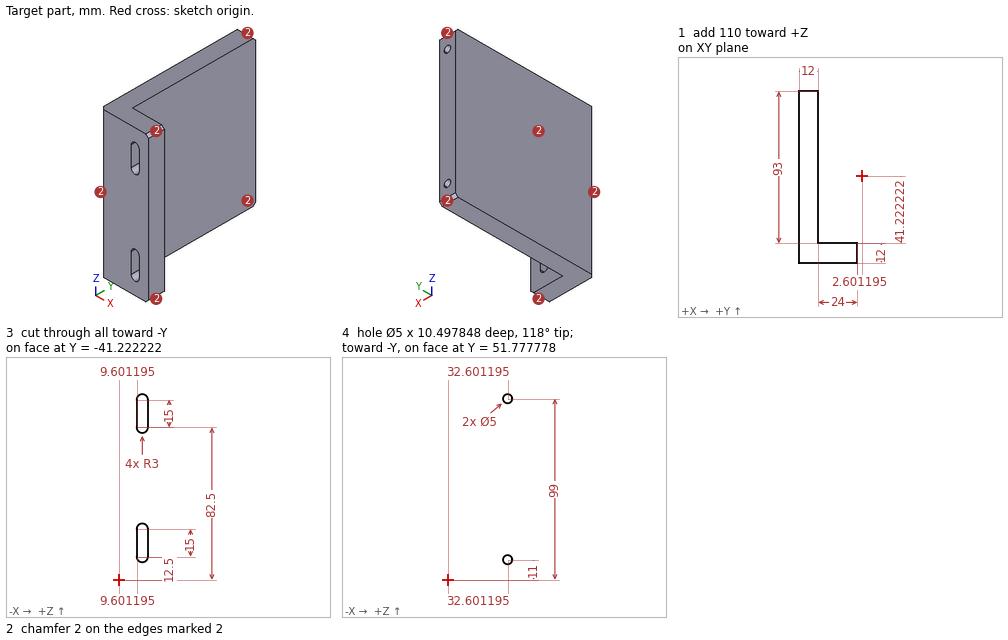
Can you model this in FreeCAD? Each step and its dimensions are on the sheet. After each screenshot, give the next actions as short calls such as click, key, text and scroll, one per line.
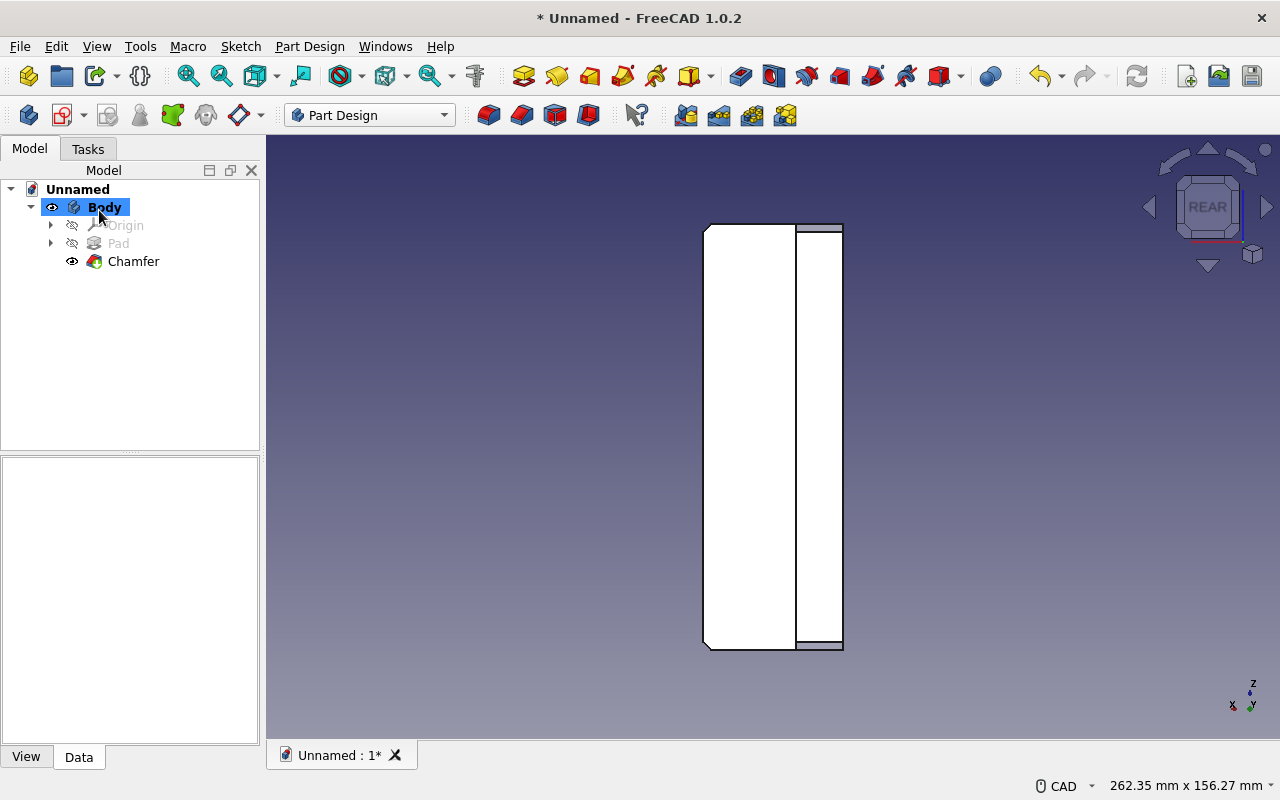
click(750, 315)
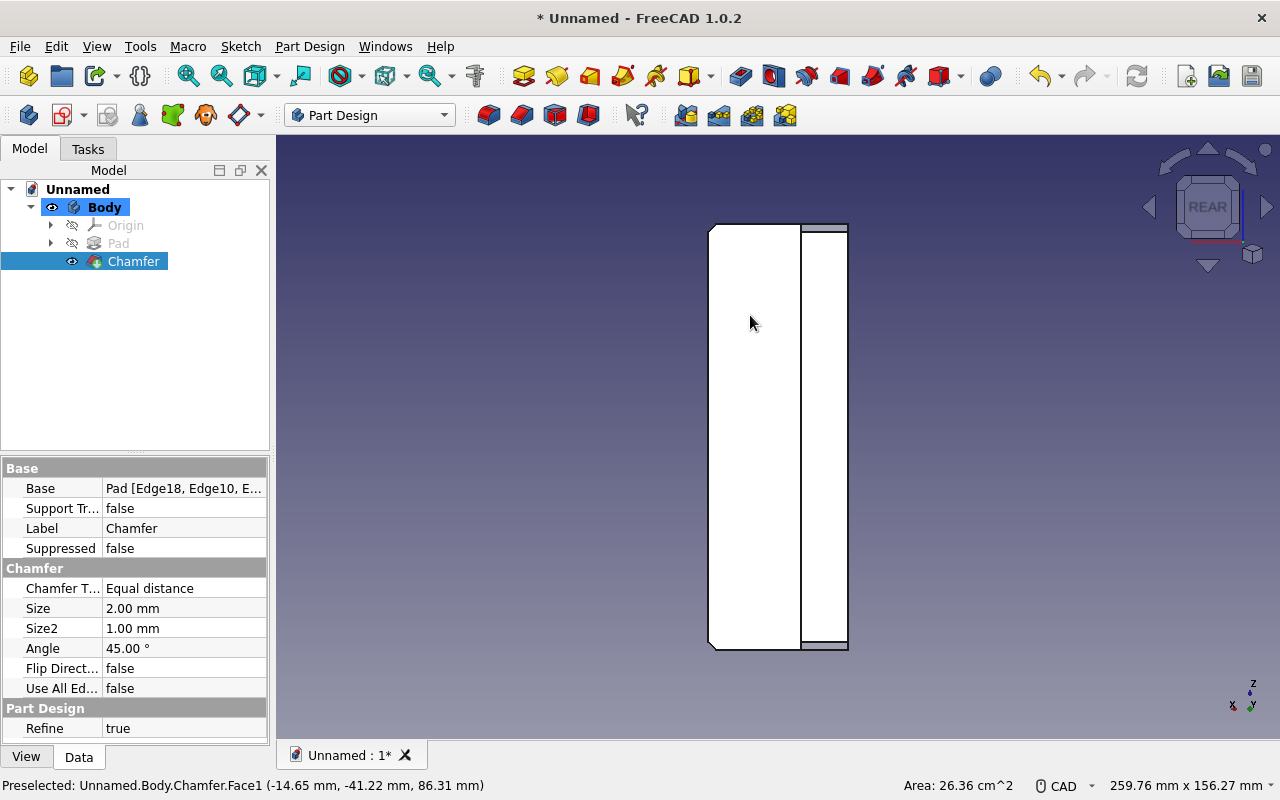
click(62, 116)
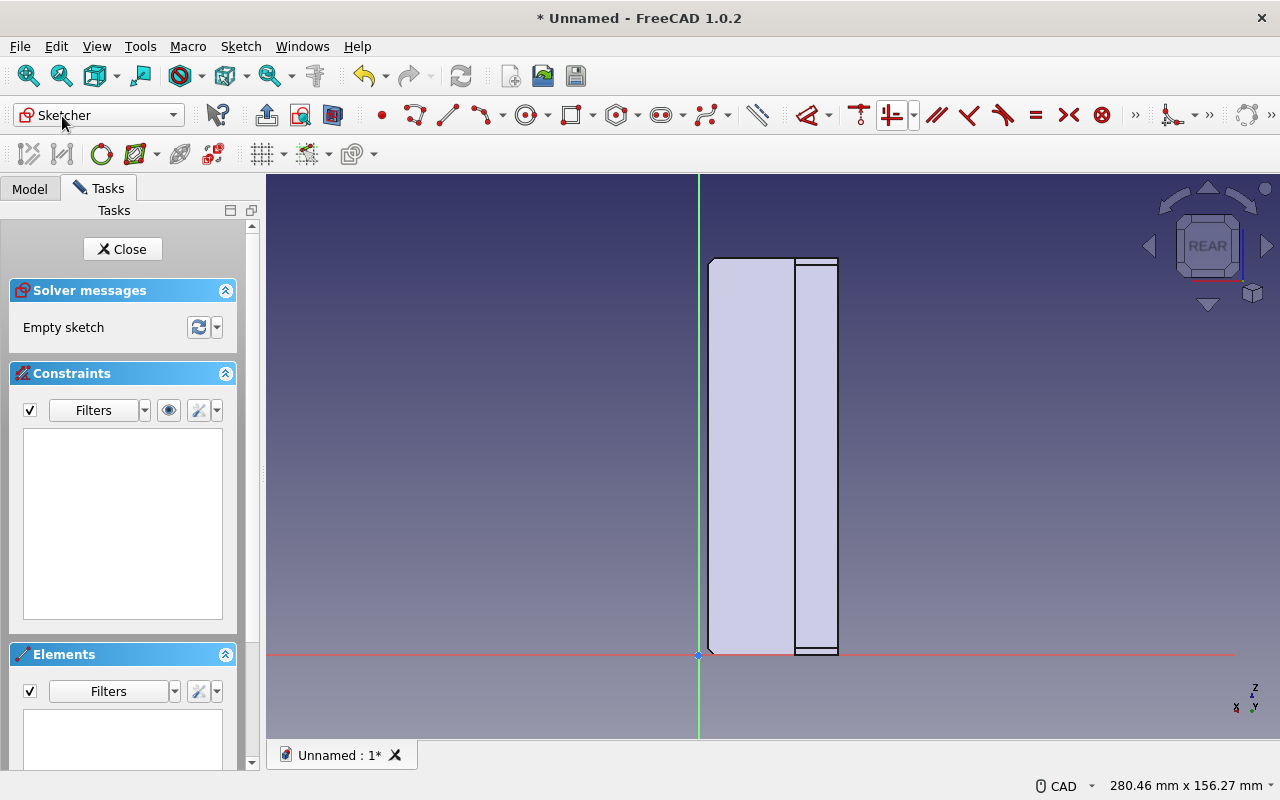
click(333, 116)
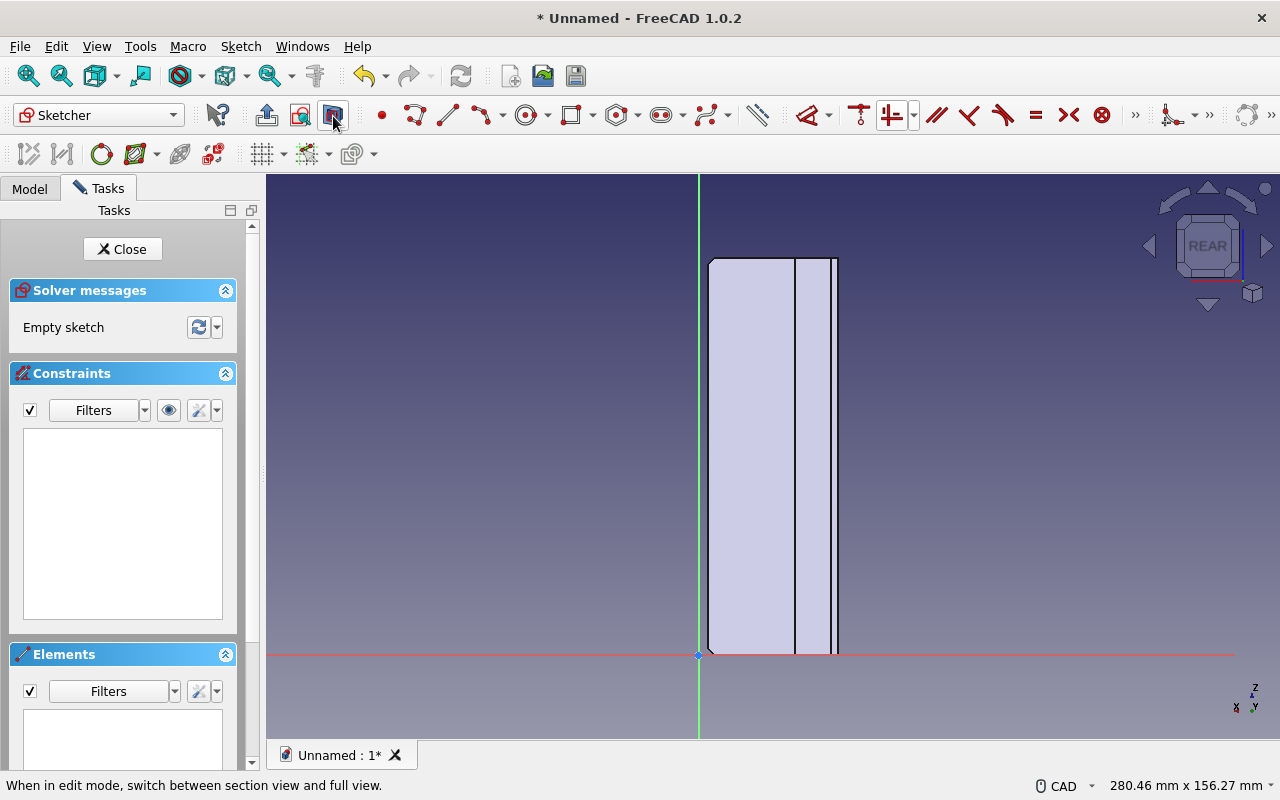
click(660, 116)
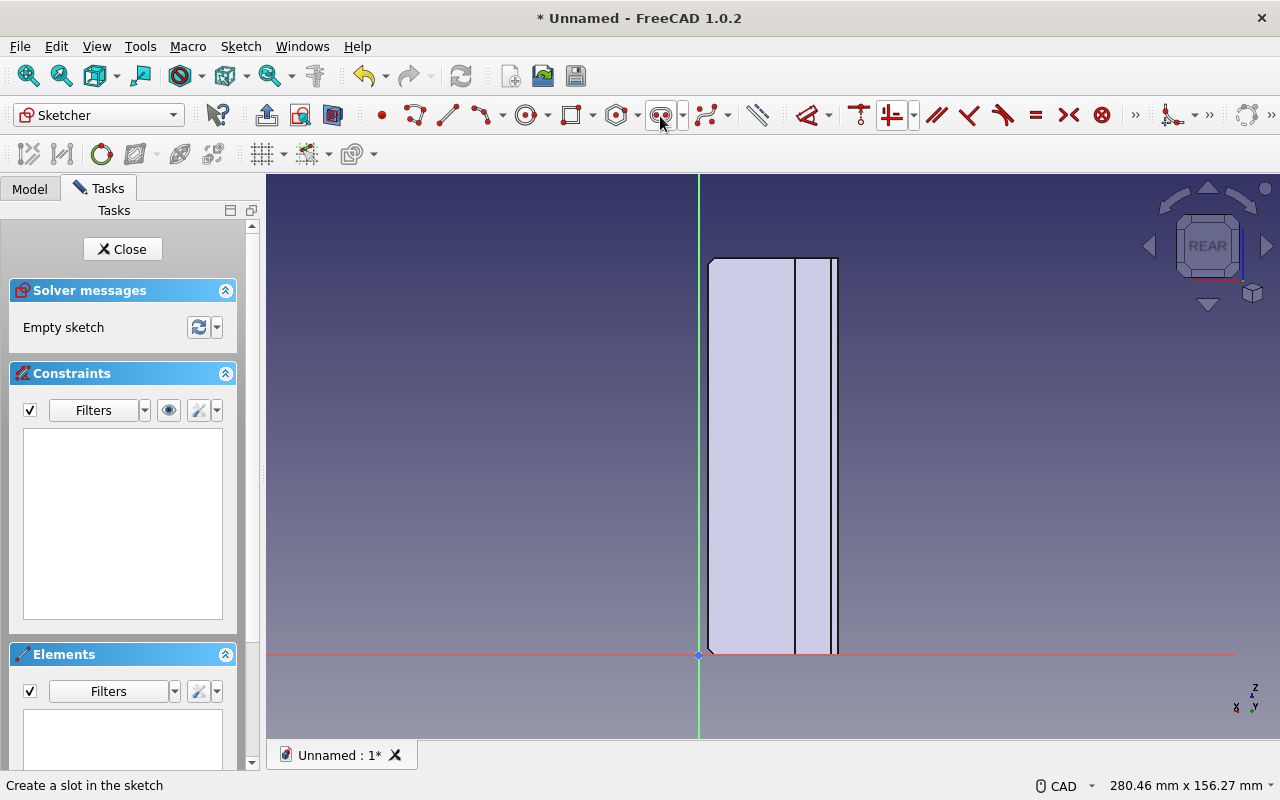
scroll(744, 357, up, 4)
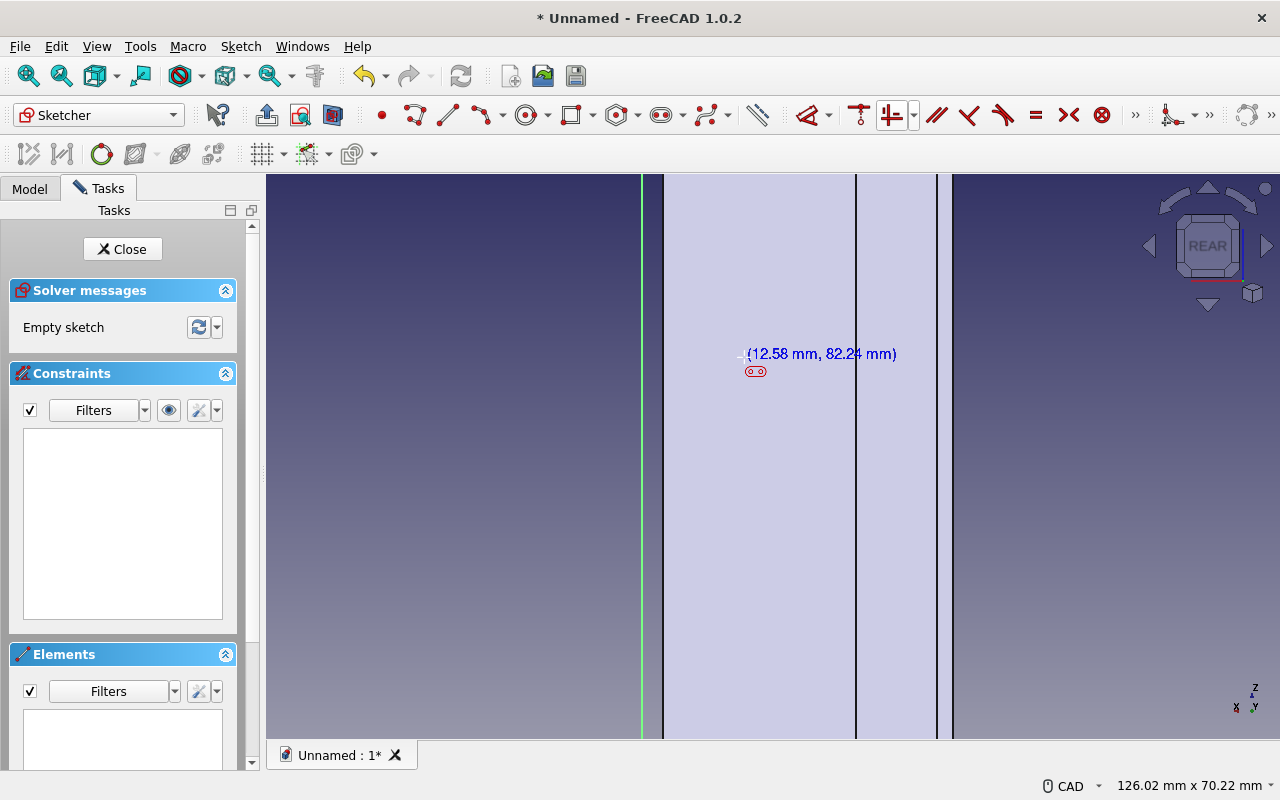
click(744, 357)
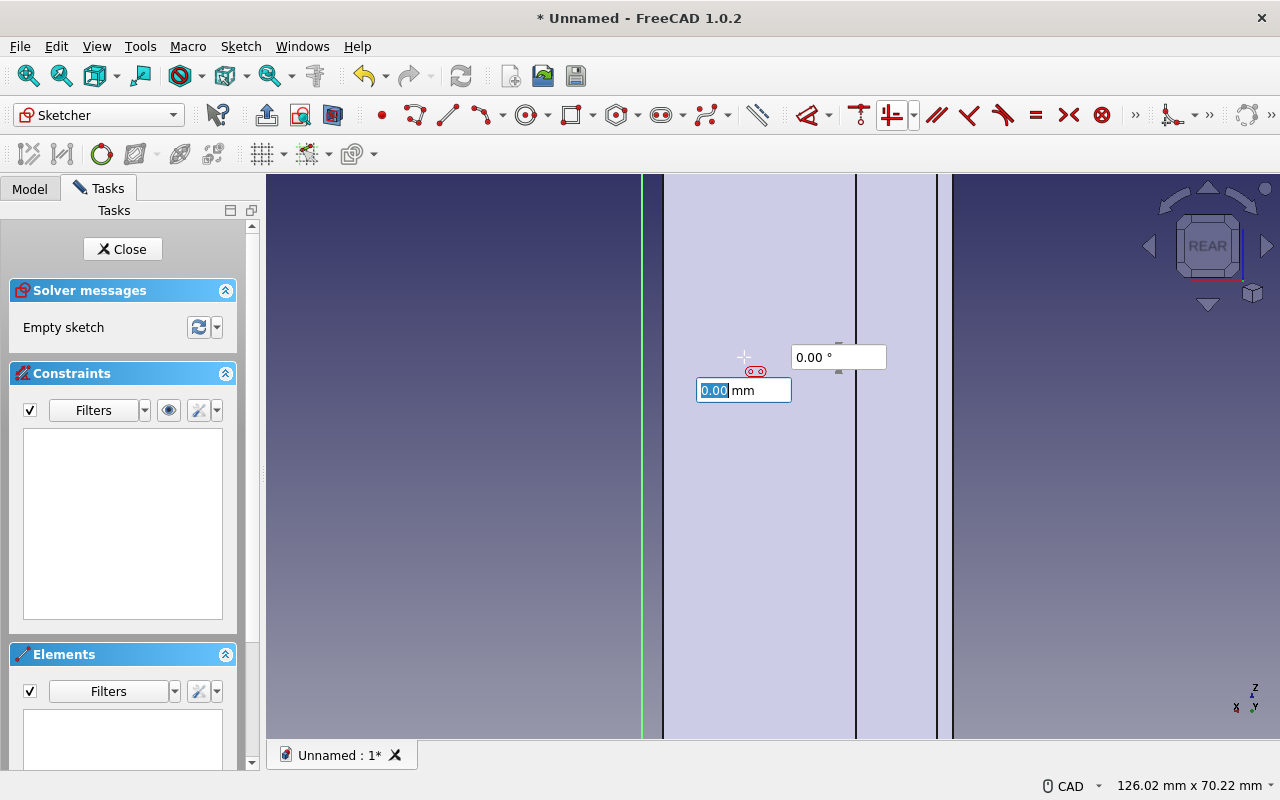
click(744, 236)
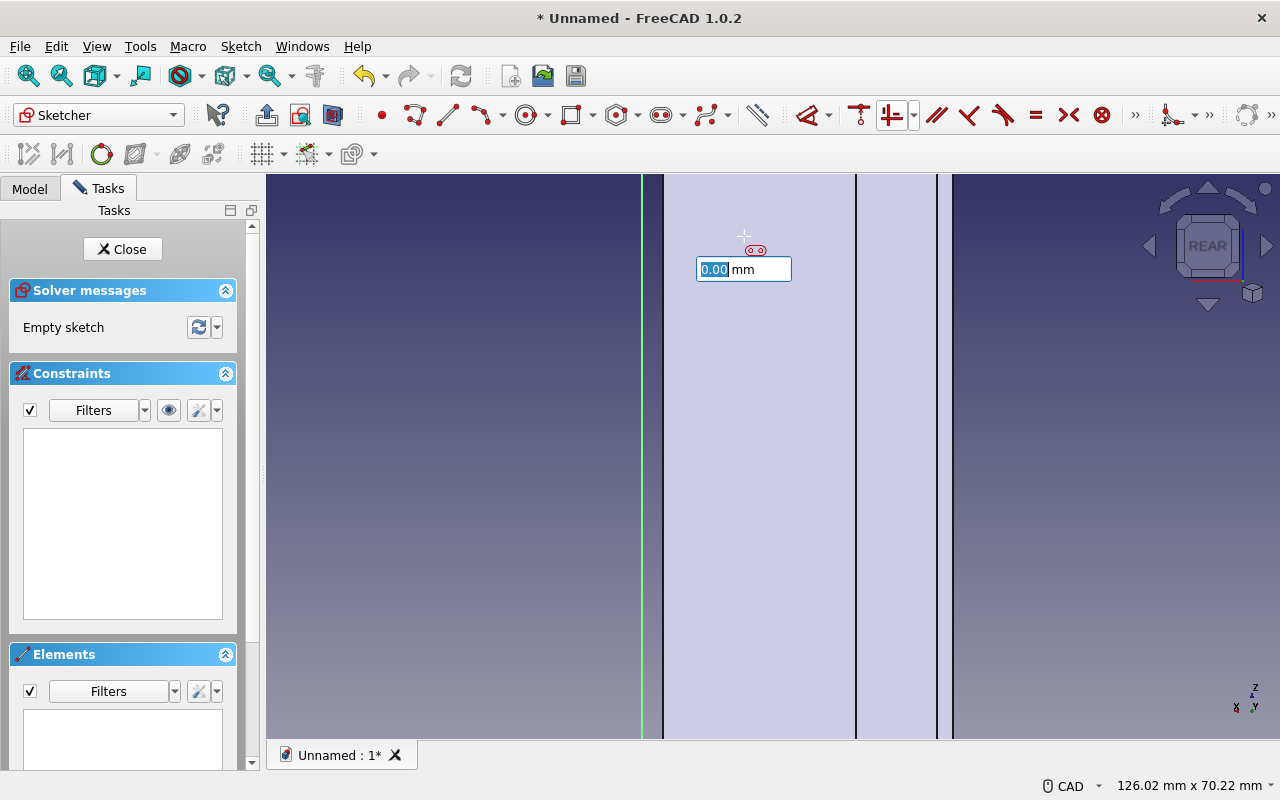
click(768, 296)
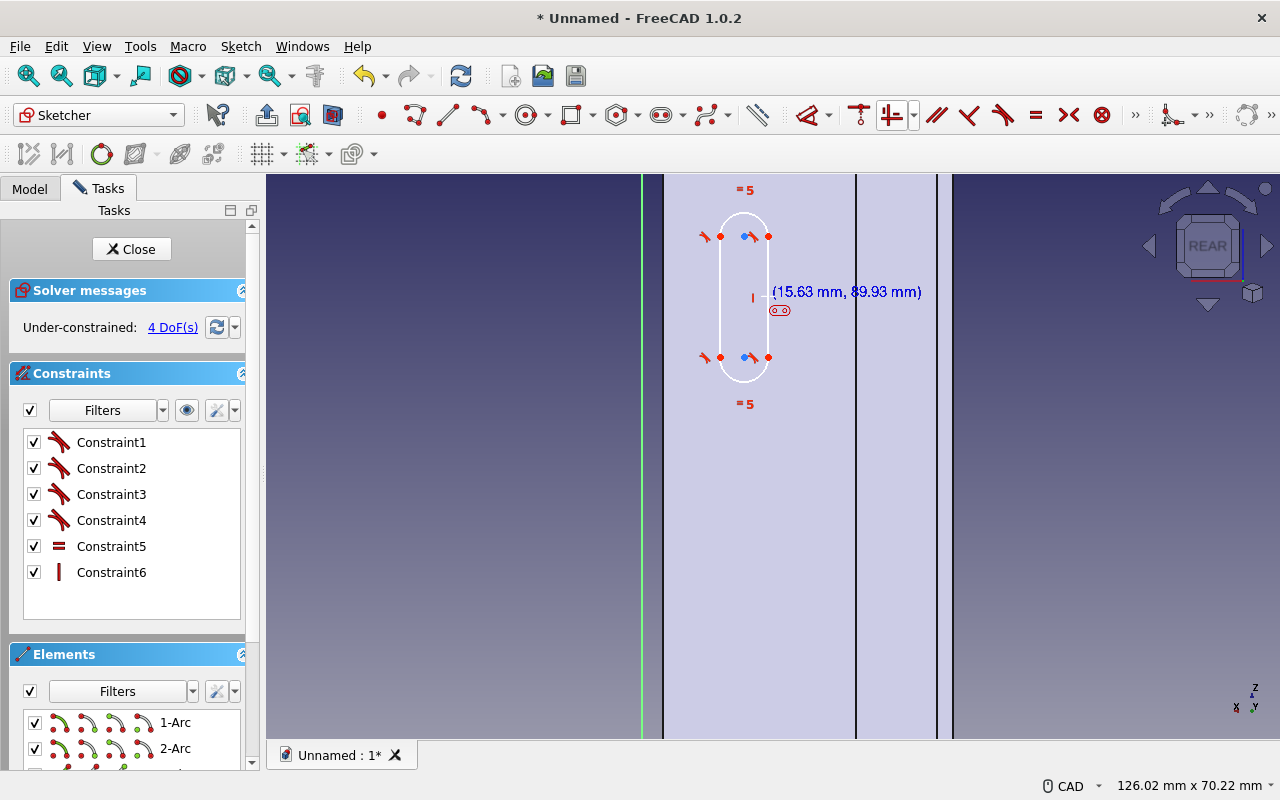
scroll(704, 326, down, 4)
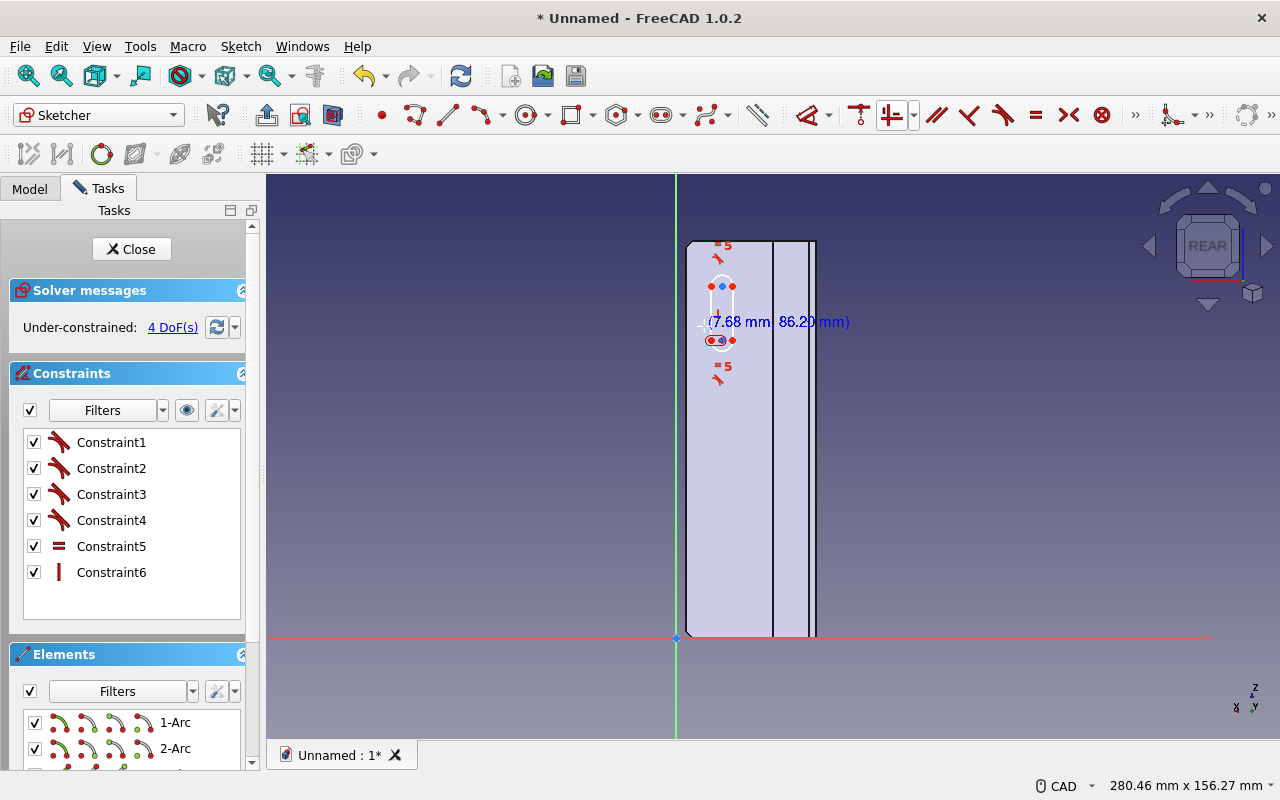
scroll(722, 593, up, 4)